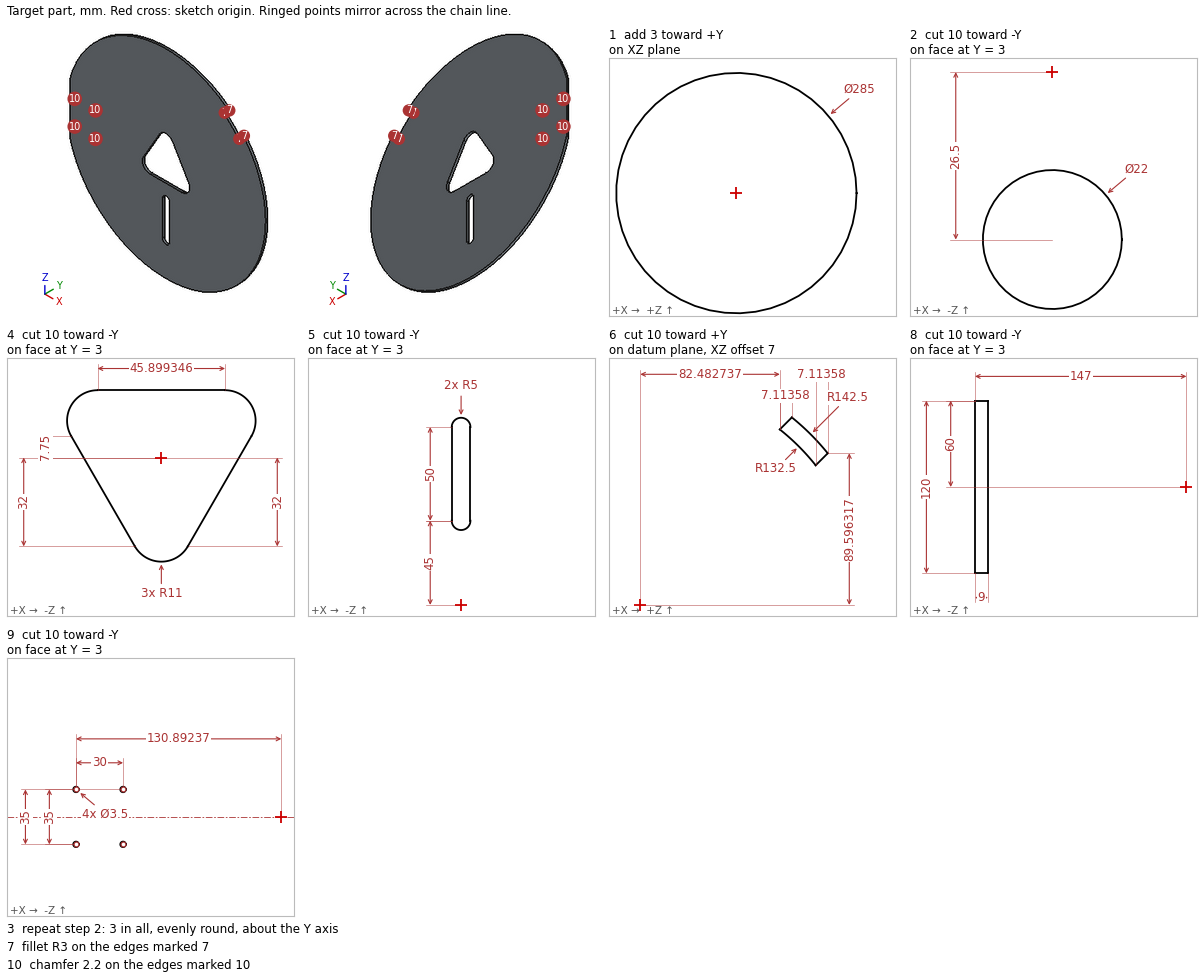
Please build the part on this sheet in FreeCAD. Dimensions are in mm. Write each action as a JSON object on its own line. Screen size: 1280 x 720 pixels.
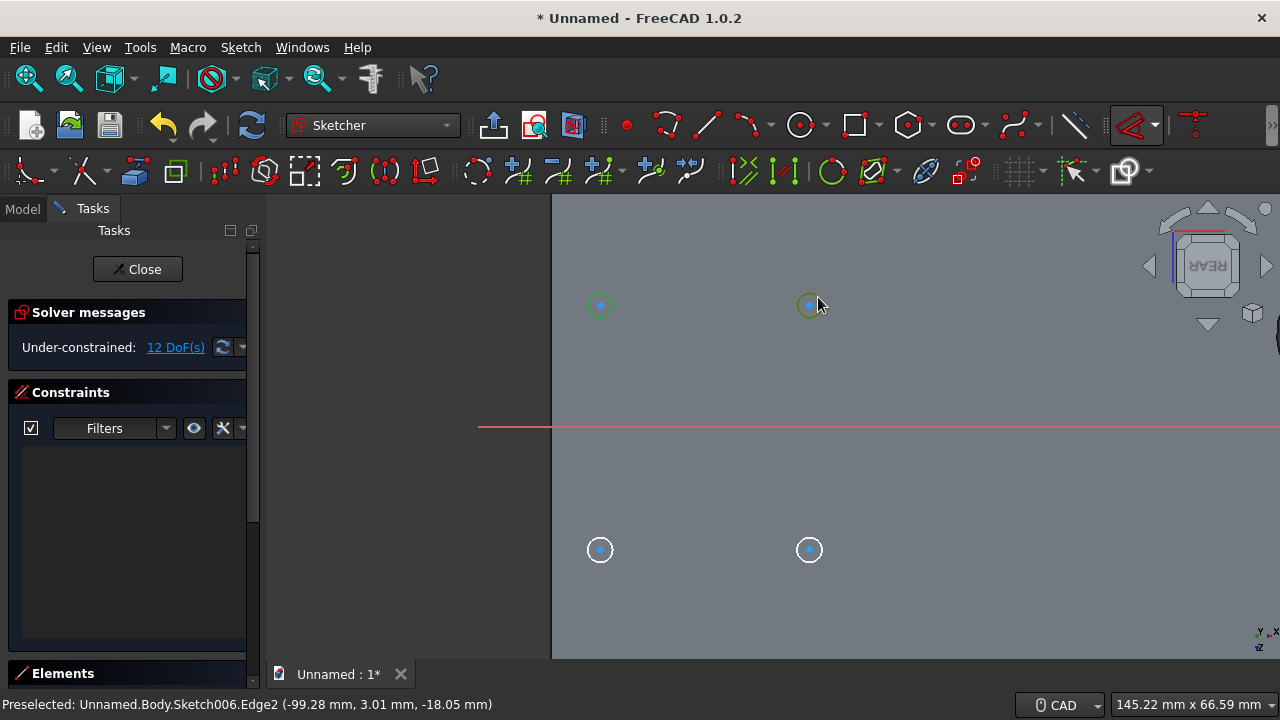
{"action": "left_click", "coordinate": [609, 541]}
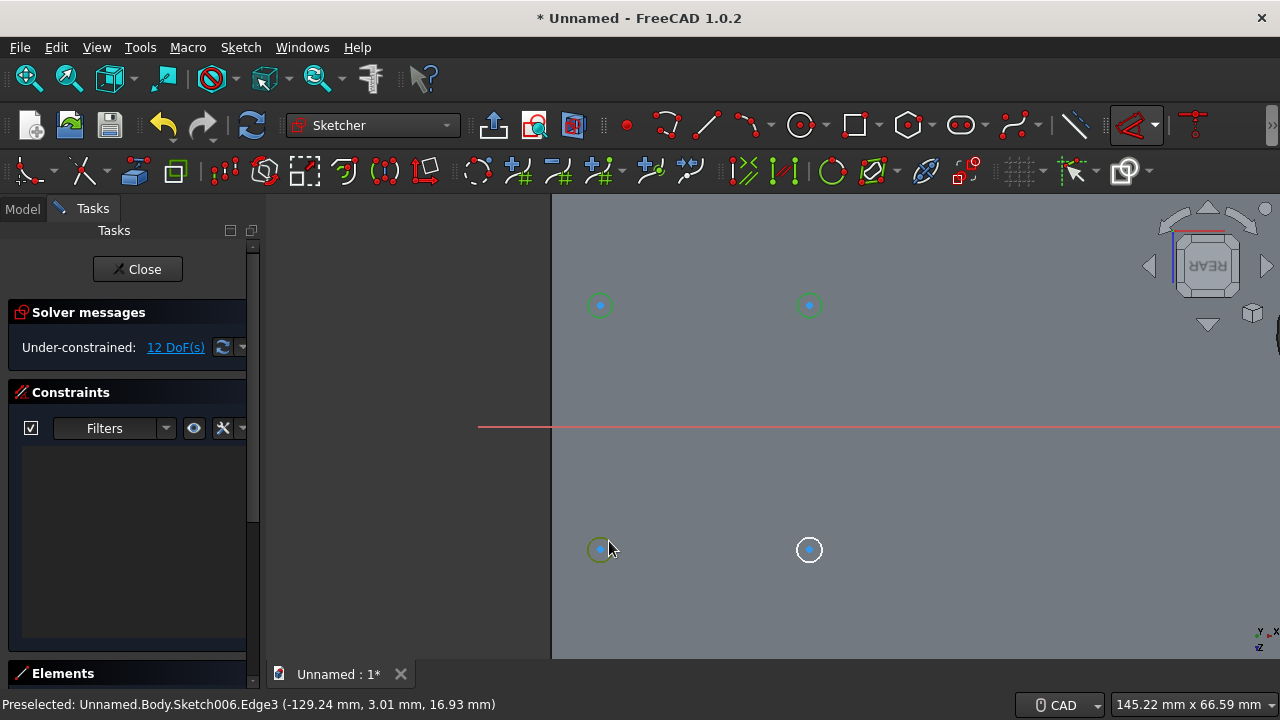
{"action": "left_click", "coordinate": [818, 541]}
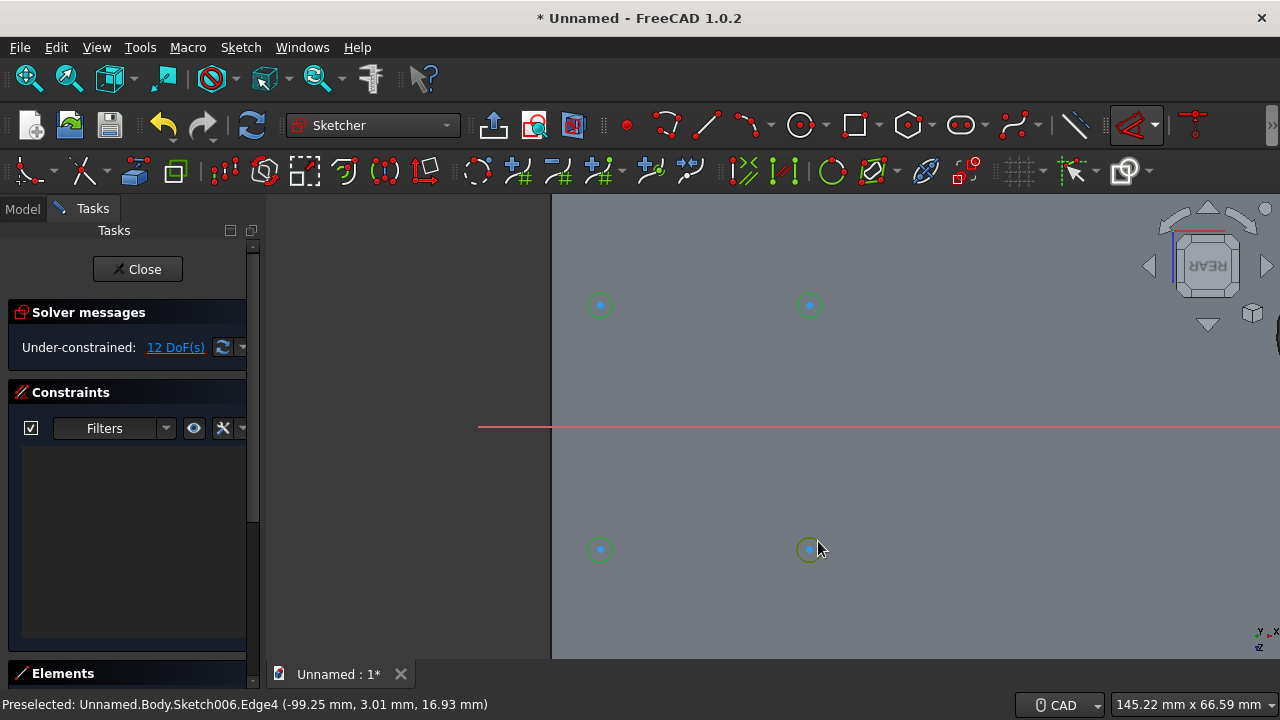
{"action": "key", "text": "e"}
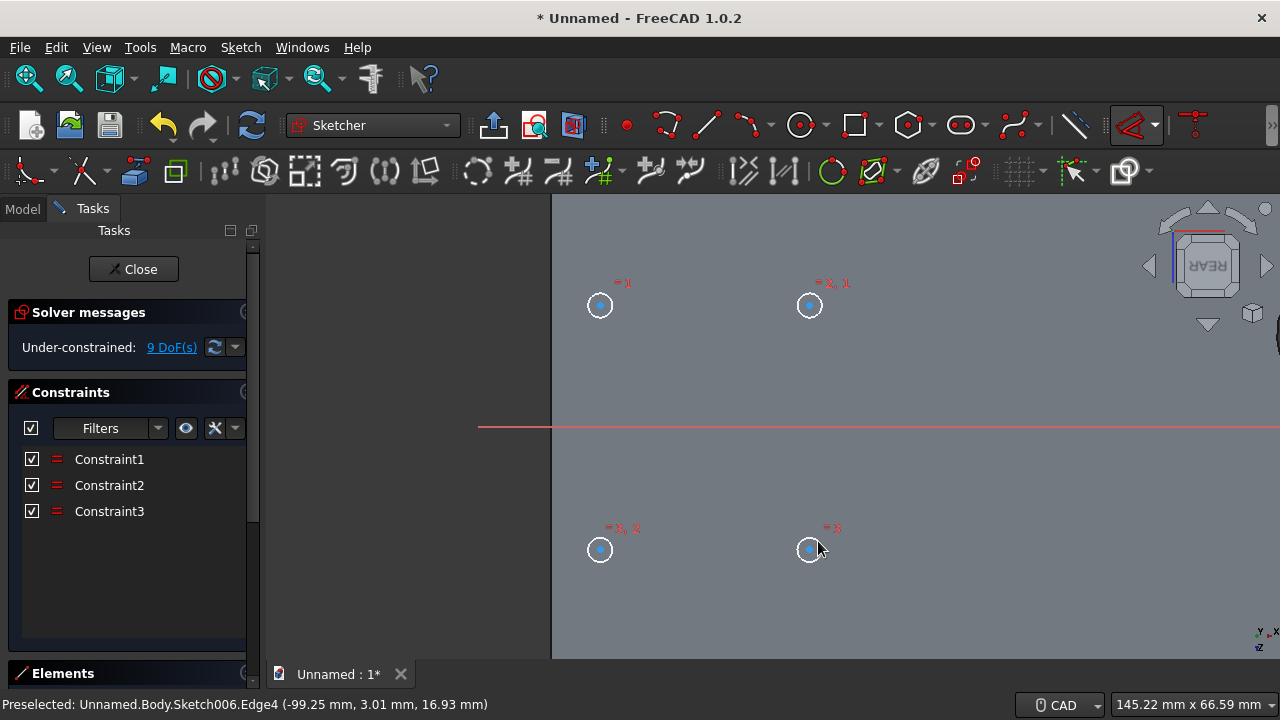
{"action": "left_click", "coordinate": [600, 306]}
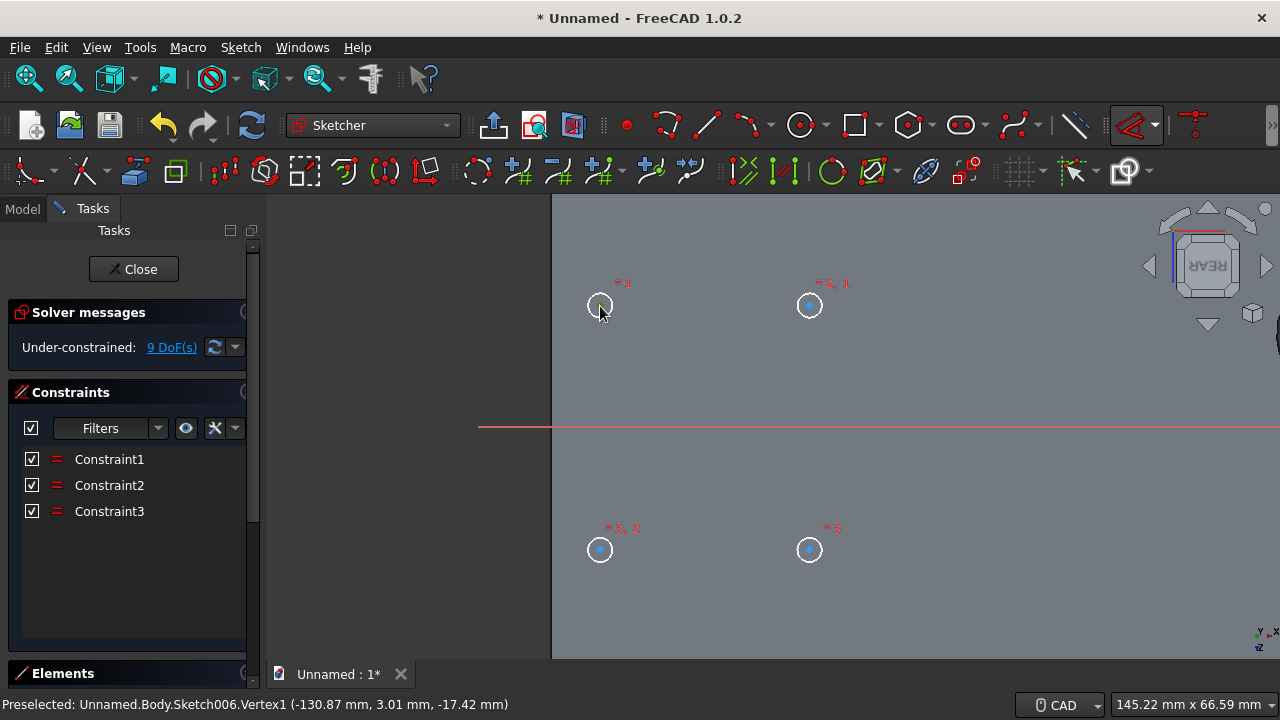
{"action": "left_click", "coordinate": [600, 550]}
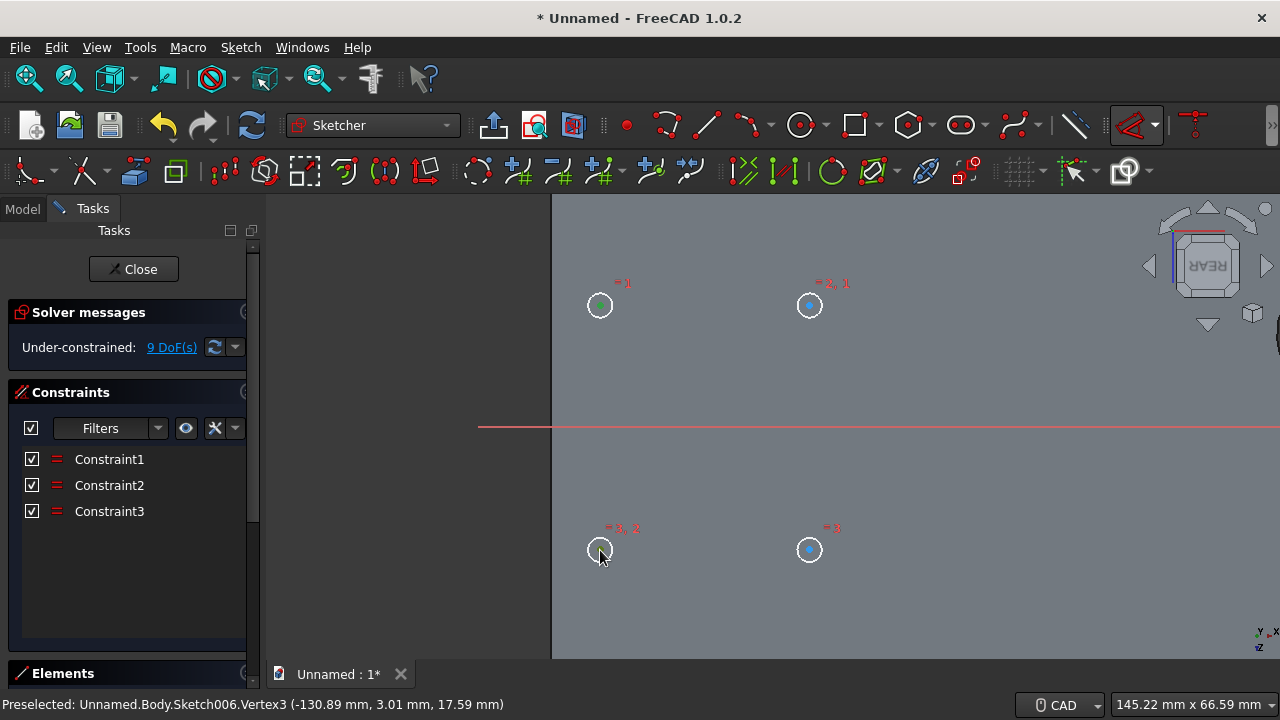
{"action": "left_click", "coordinate": [529, 427]}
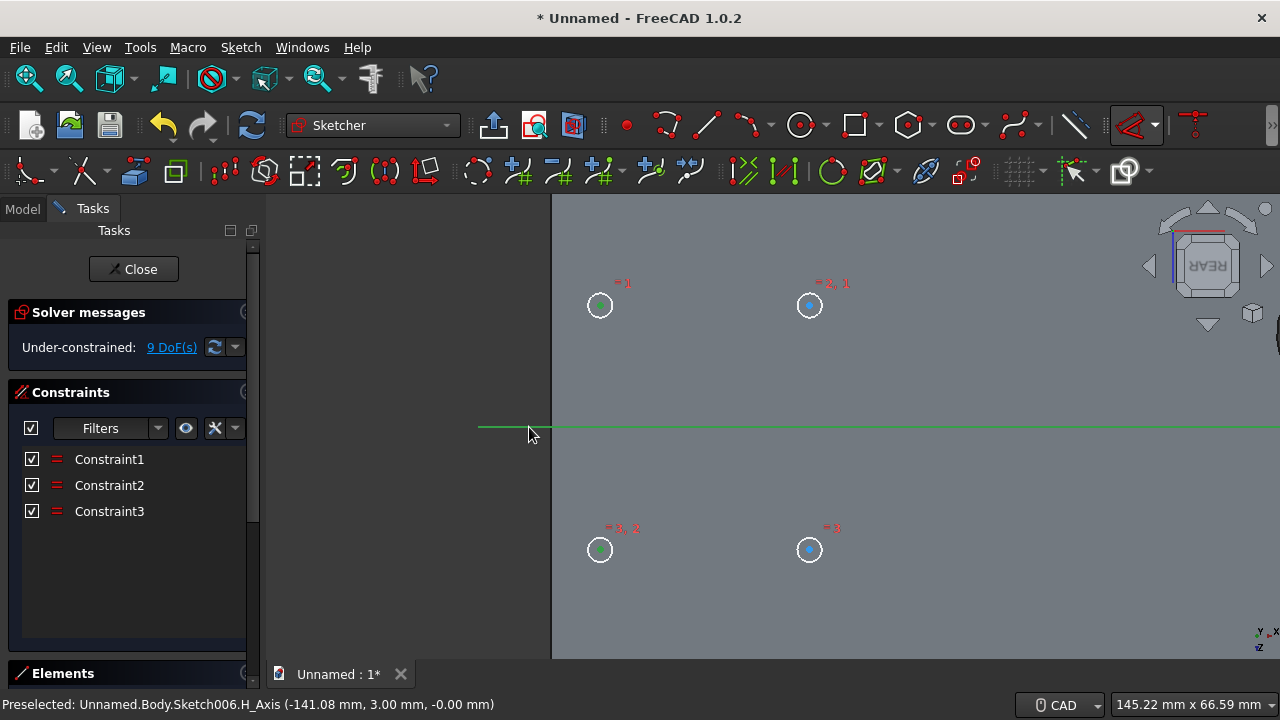
{"action": "key", "text": "s"}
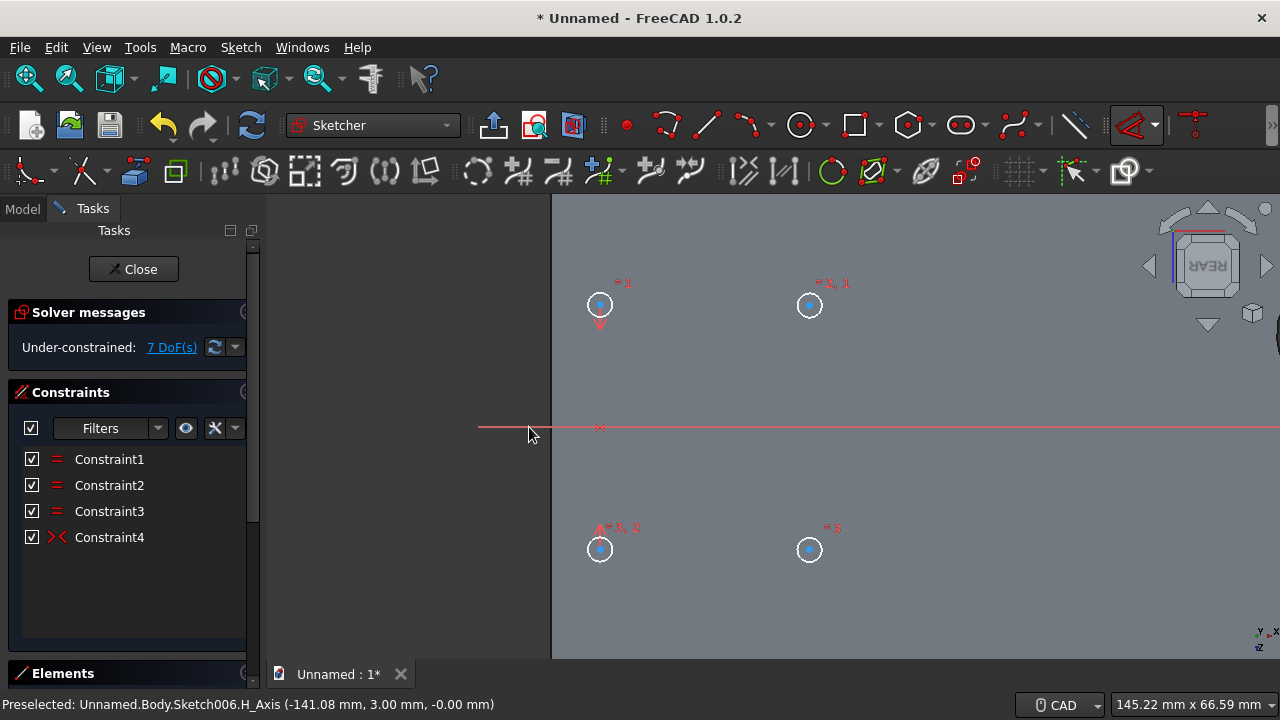
{"action": "left_click", "coordinate": [810, 306]}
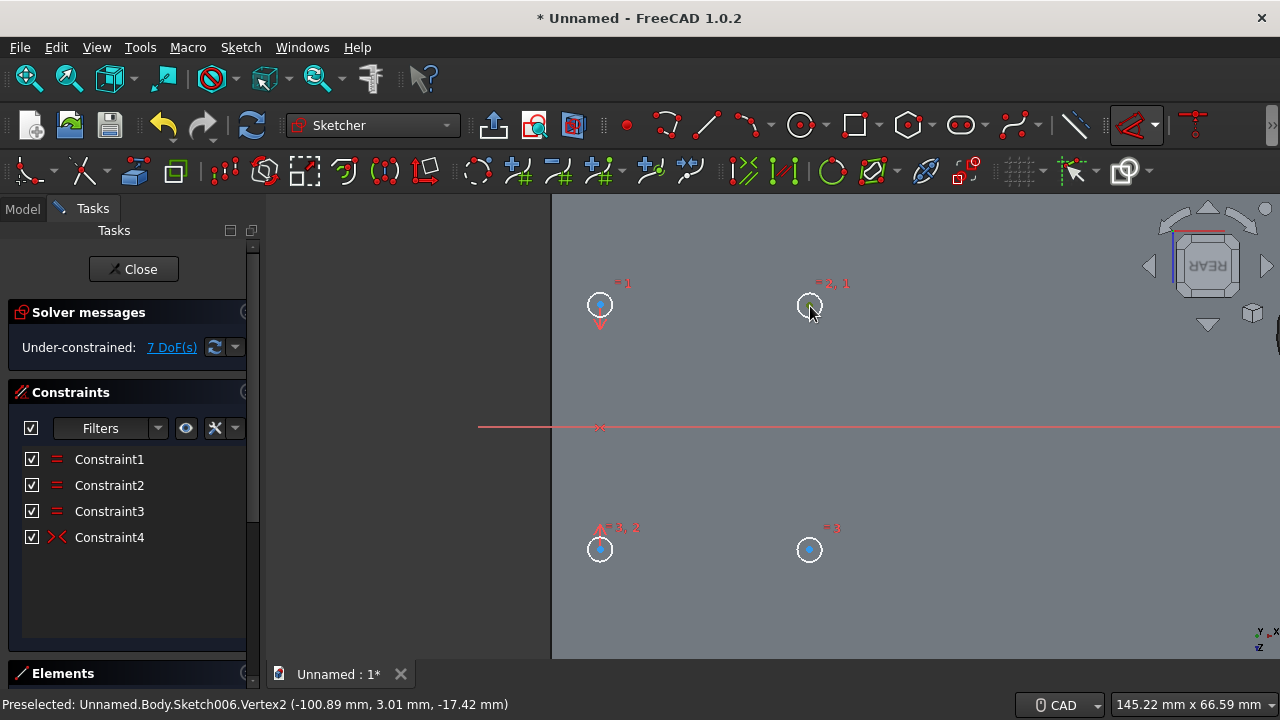
{"action": "left_click", "coordinate": [810, 550]}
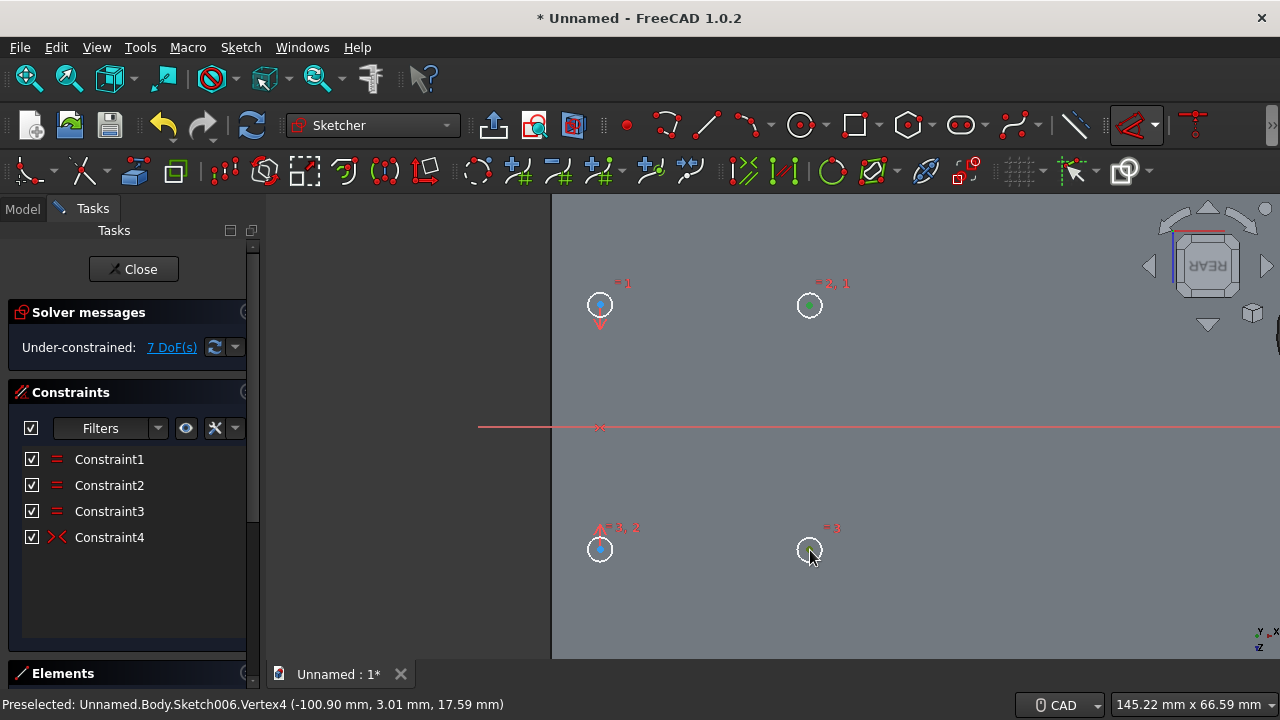
{"action": "left_click", "coordinate": [529, 427]}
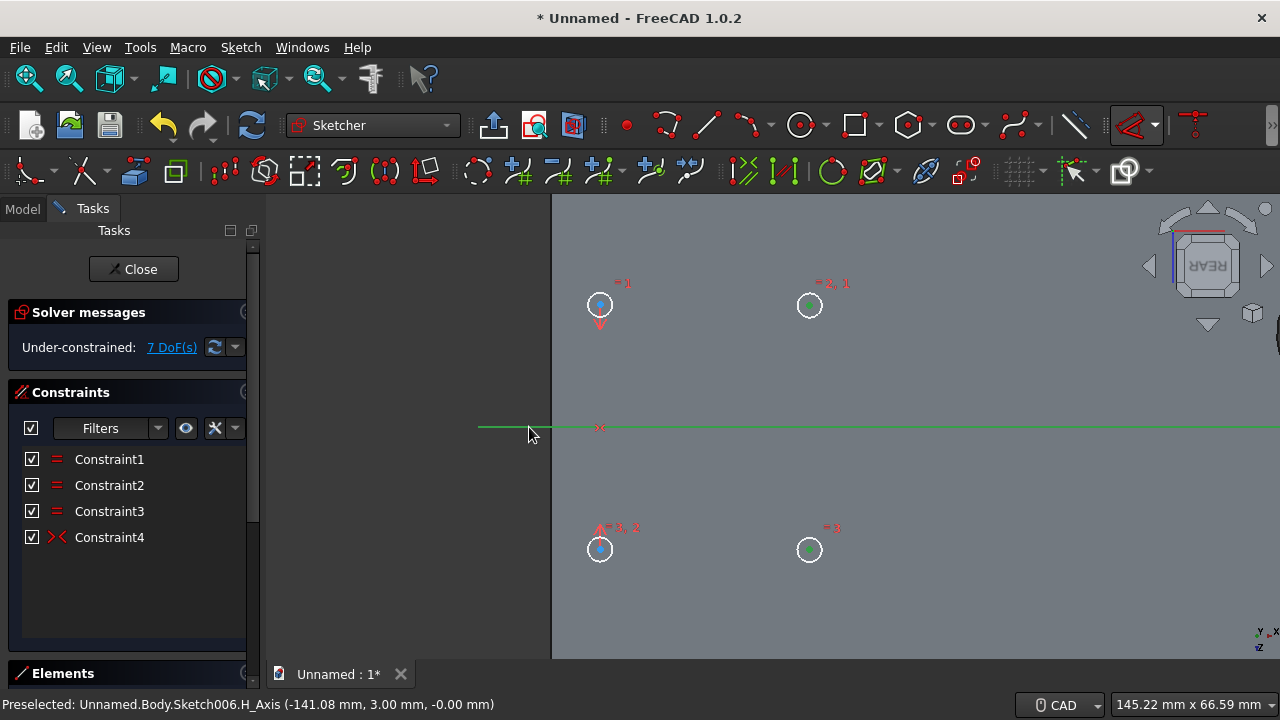
{"action": "key", "text": "s"}